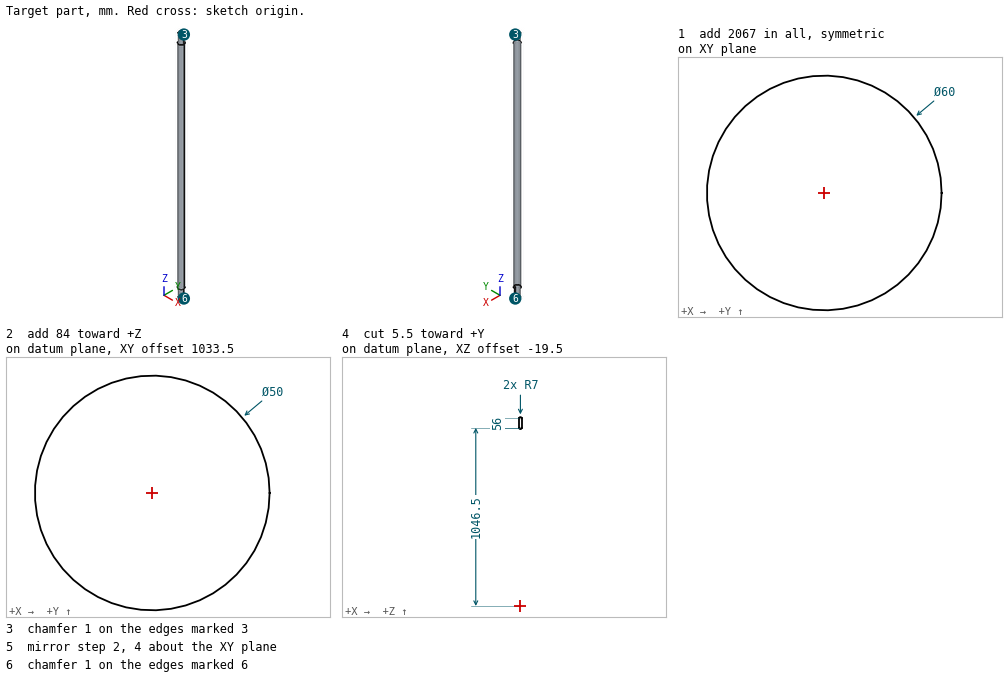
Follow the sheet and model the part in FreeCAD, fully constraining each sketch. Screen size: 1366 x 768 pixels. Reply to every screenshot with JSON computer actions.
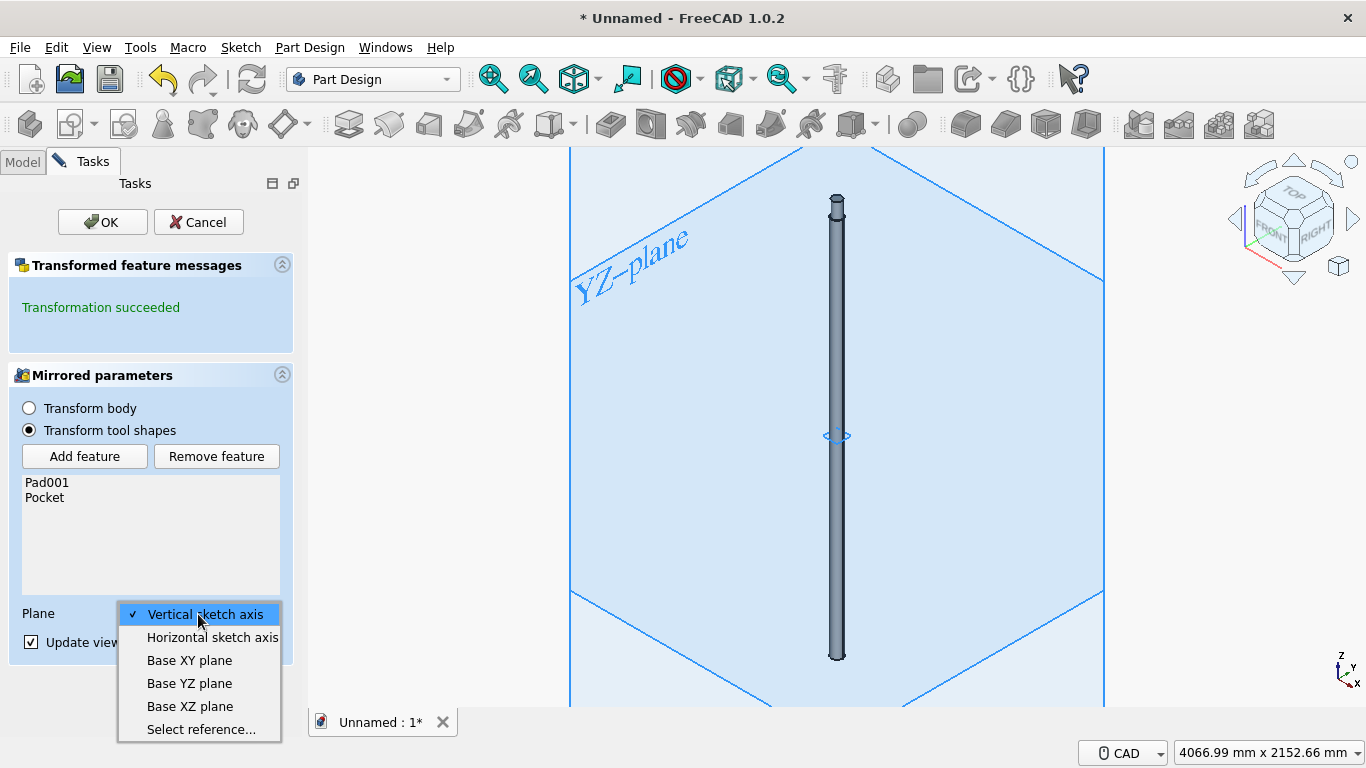
{"action": "left_click", "coordinate": [198, 660]}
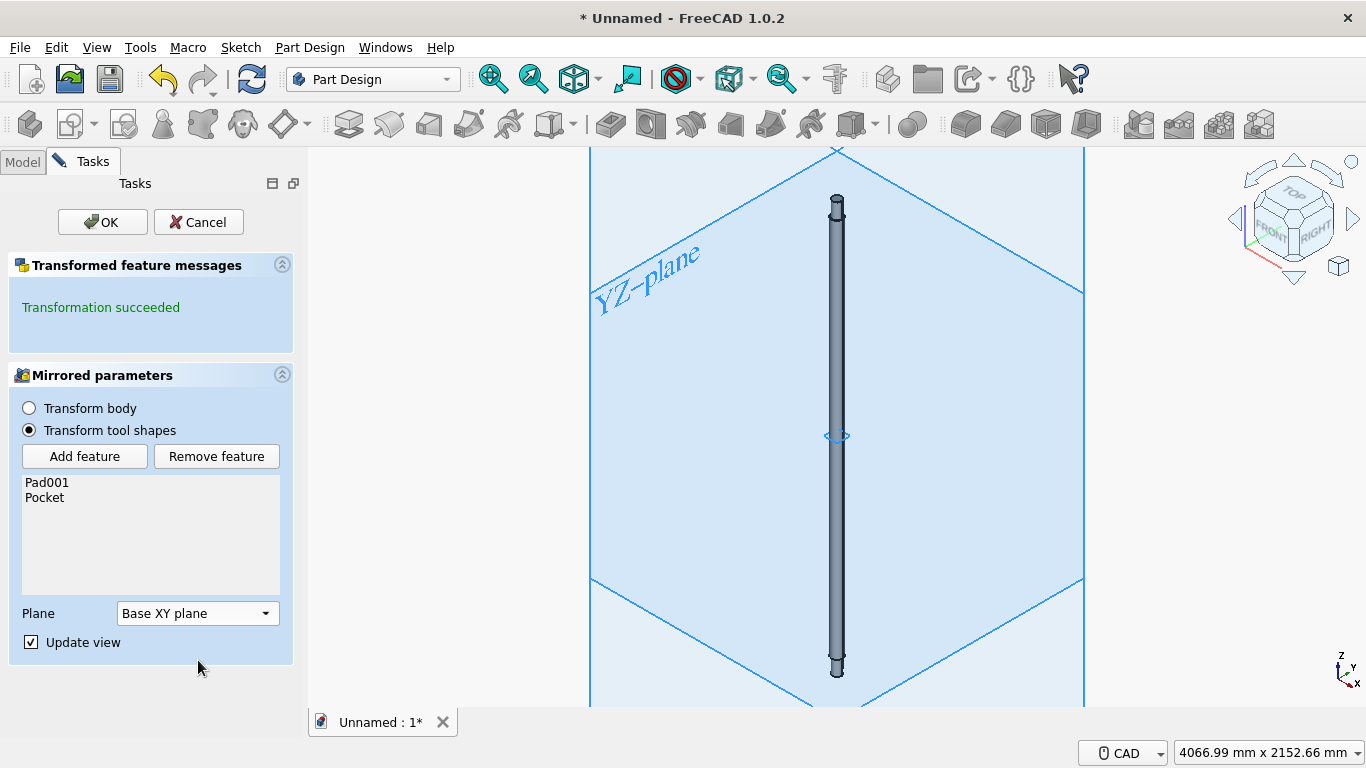
{"action": "left_click", "coordinate": [103, 222]}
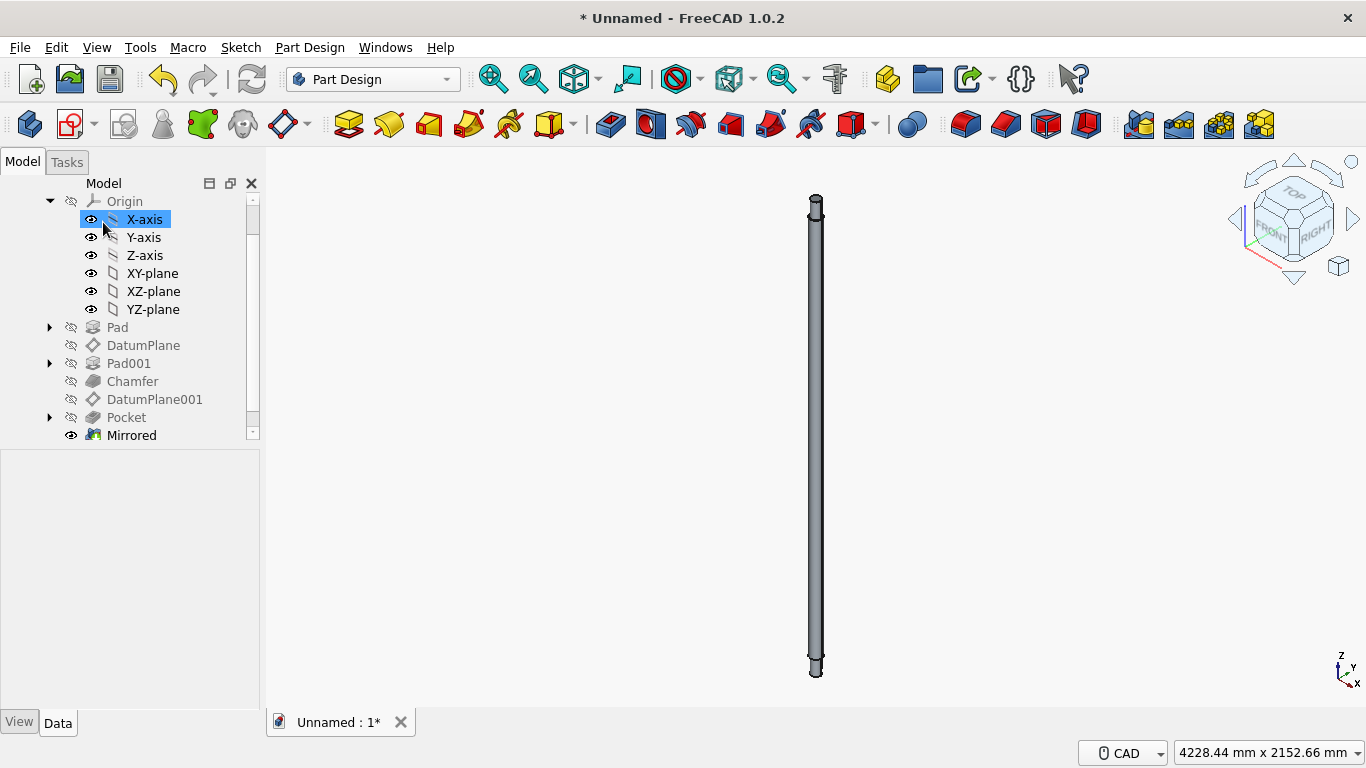
{"action": "left_click", "coordinate": [810, 674]}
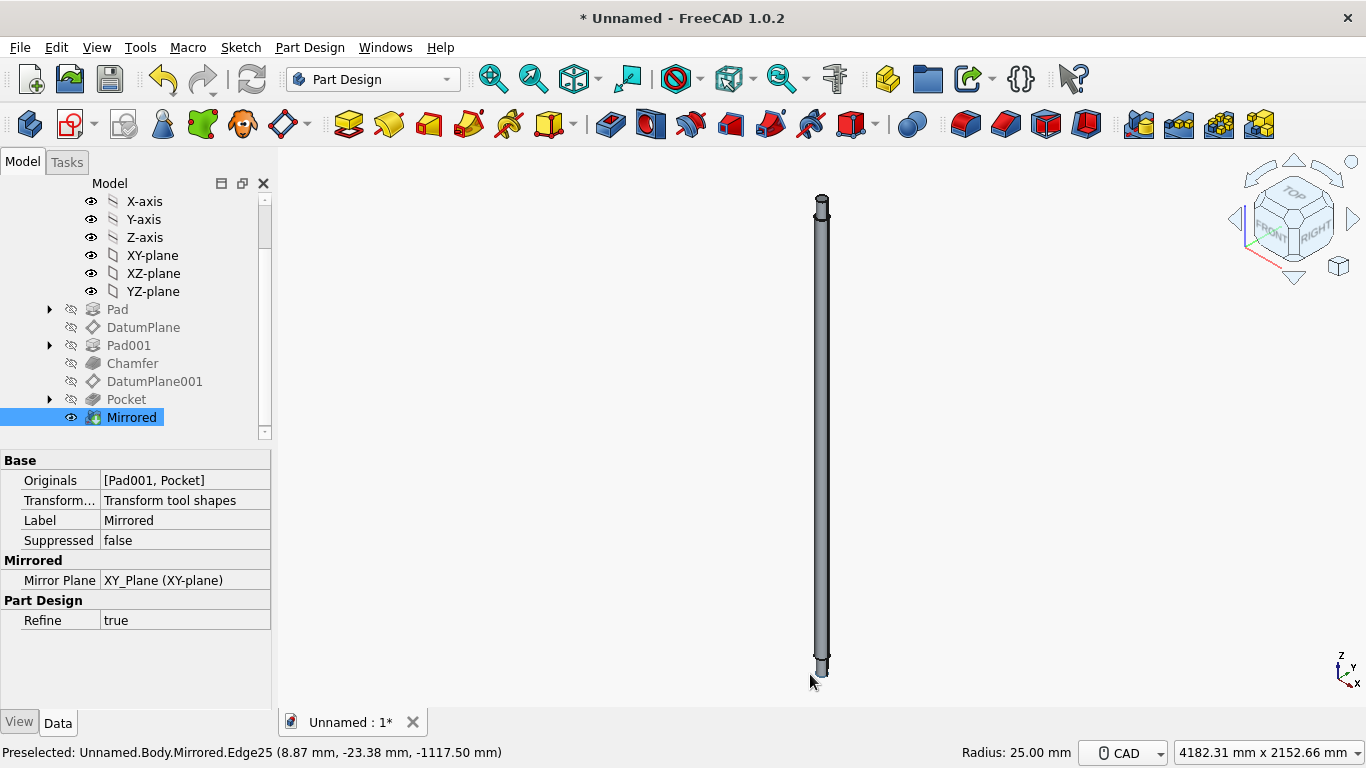
{"action": "left_click", "coordinate": [1006, 124]}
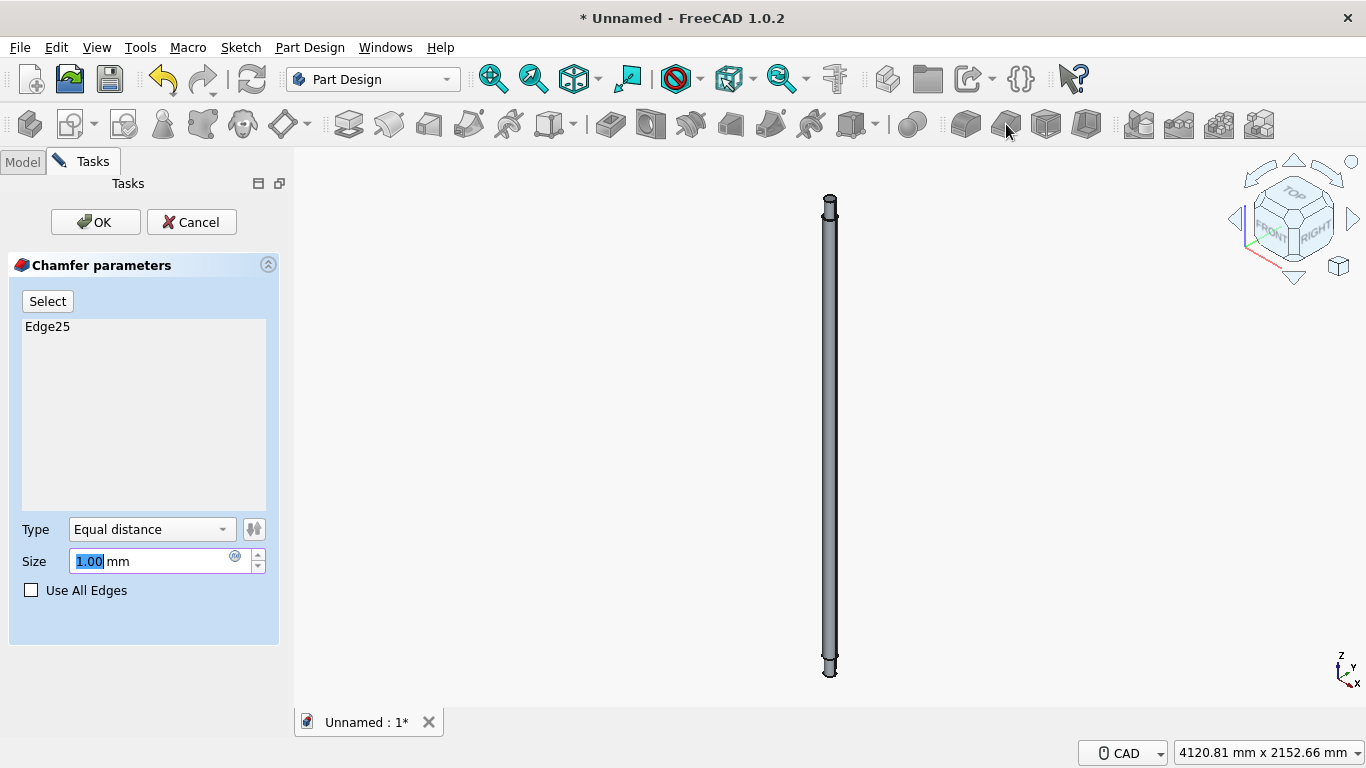
{"action": "type", "text": "1"}
{"action": "key", "text": "Tab"}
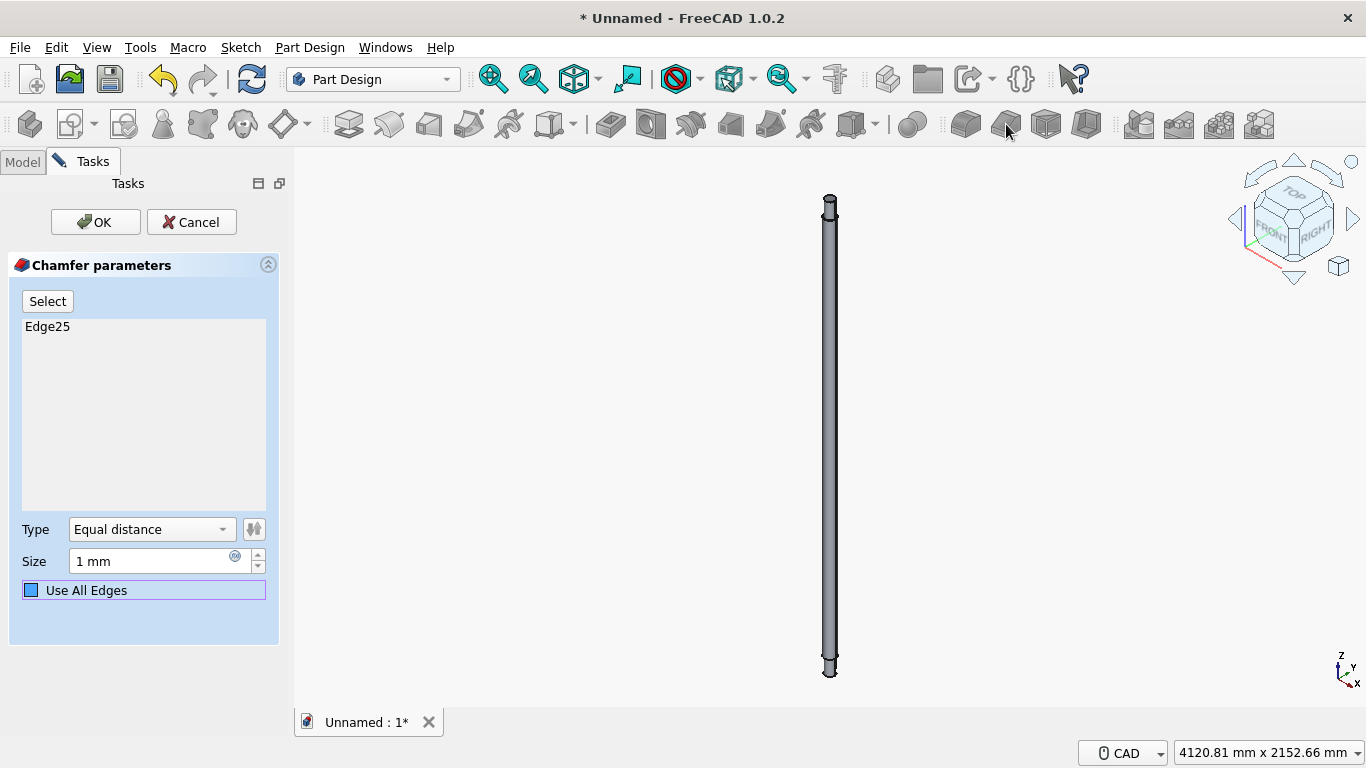
{"action": "left_click", "coordinate": [96, 222]}